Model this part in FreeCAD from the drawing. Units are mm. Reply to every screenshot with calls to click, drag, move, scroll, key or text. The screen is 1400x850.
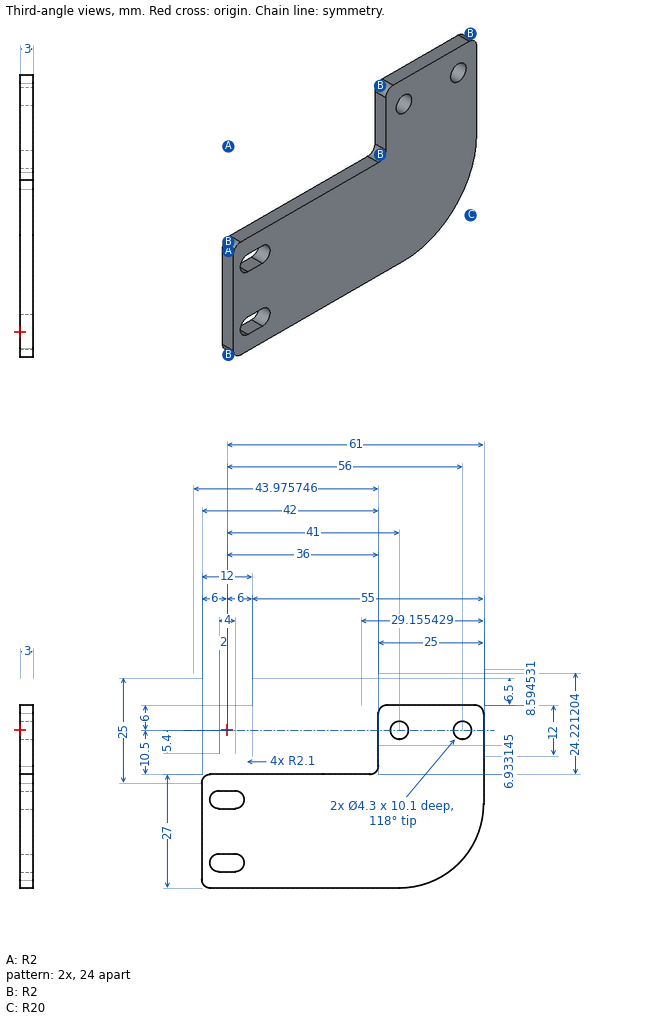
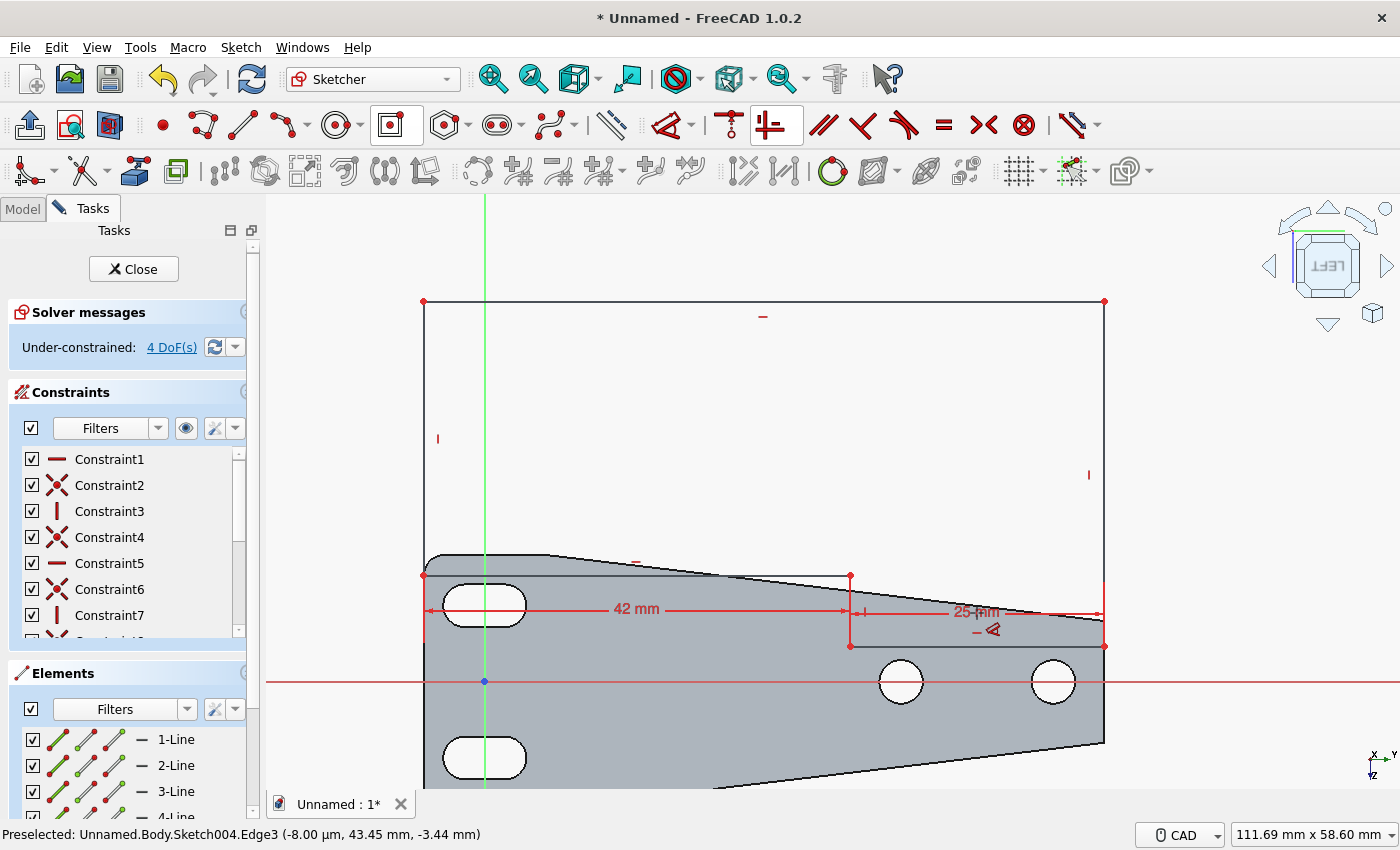
click(424, 384)
click(390, 439)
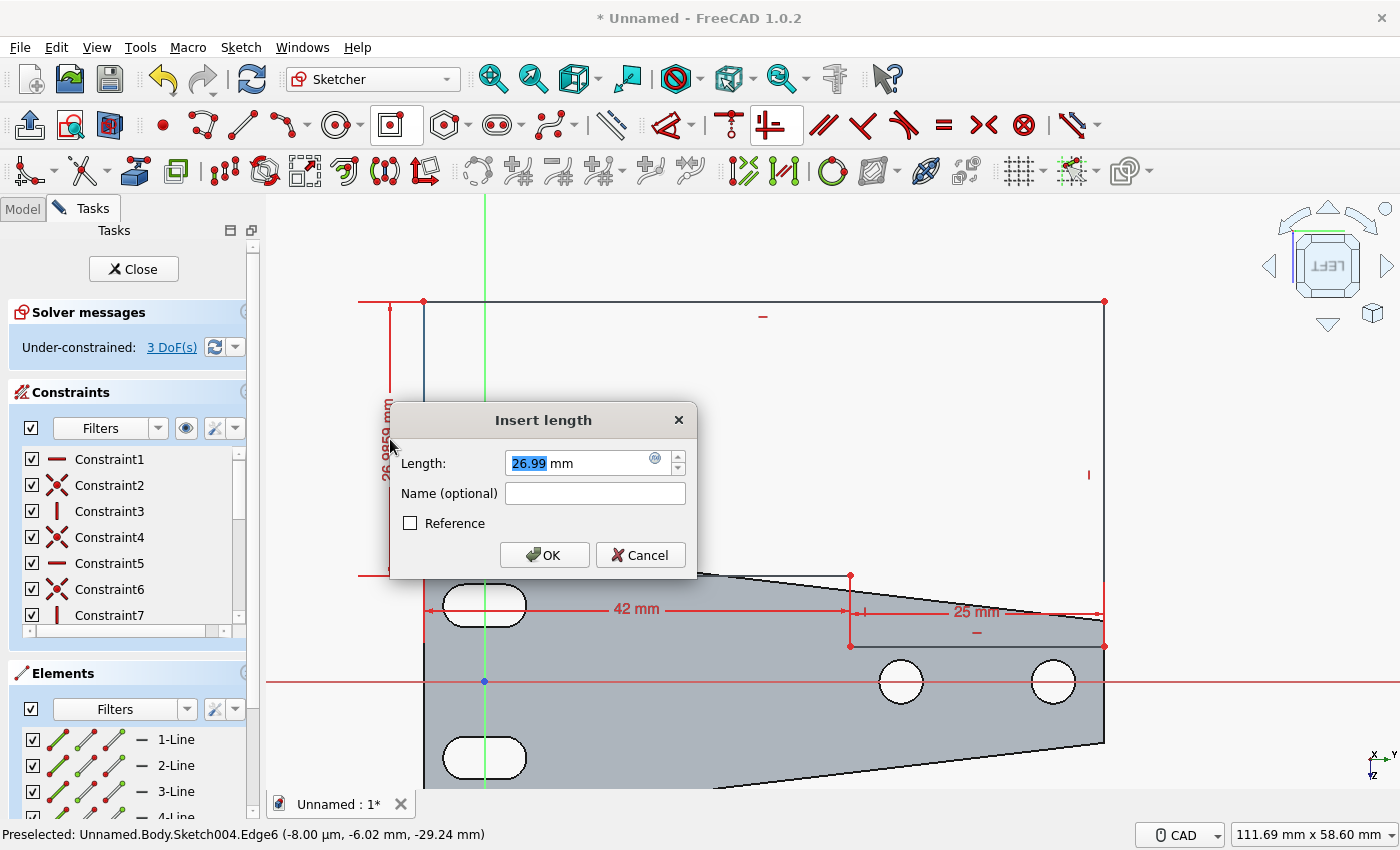
text(27)
key(Return)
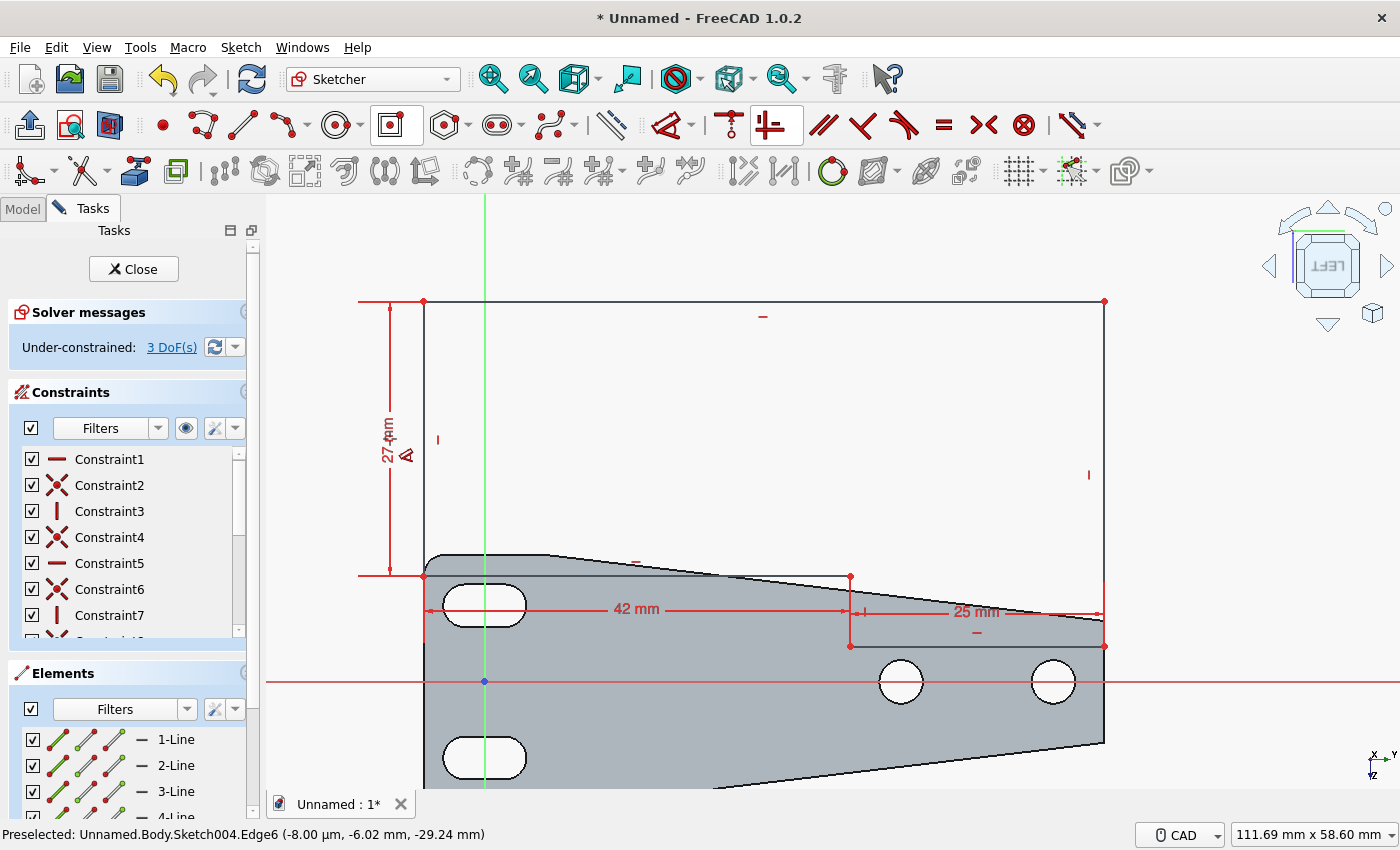
click(424, 576)
click(454, 716)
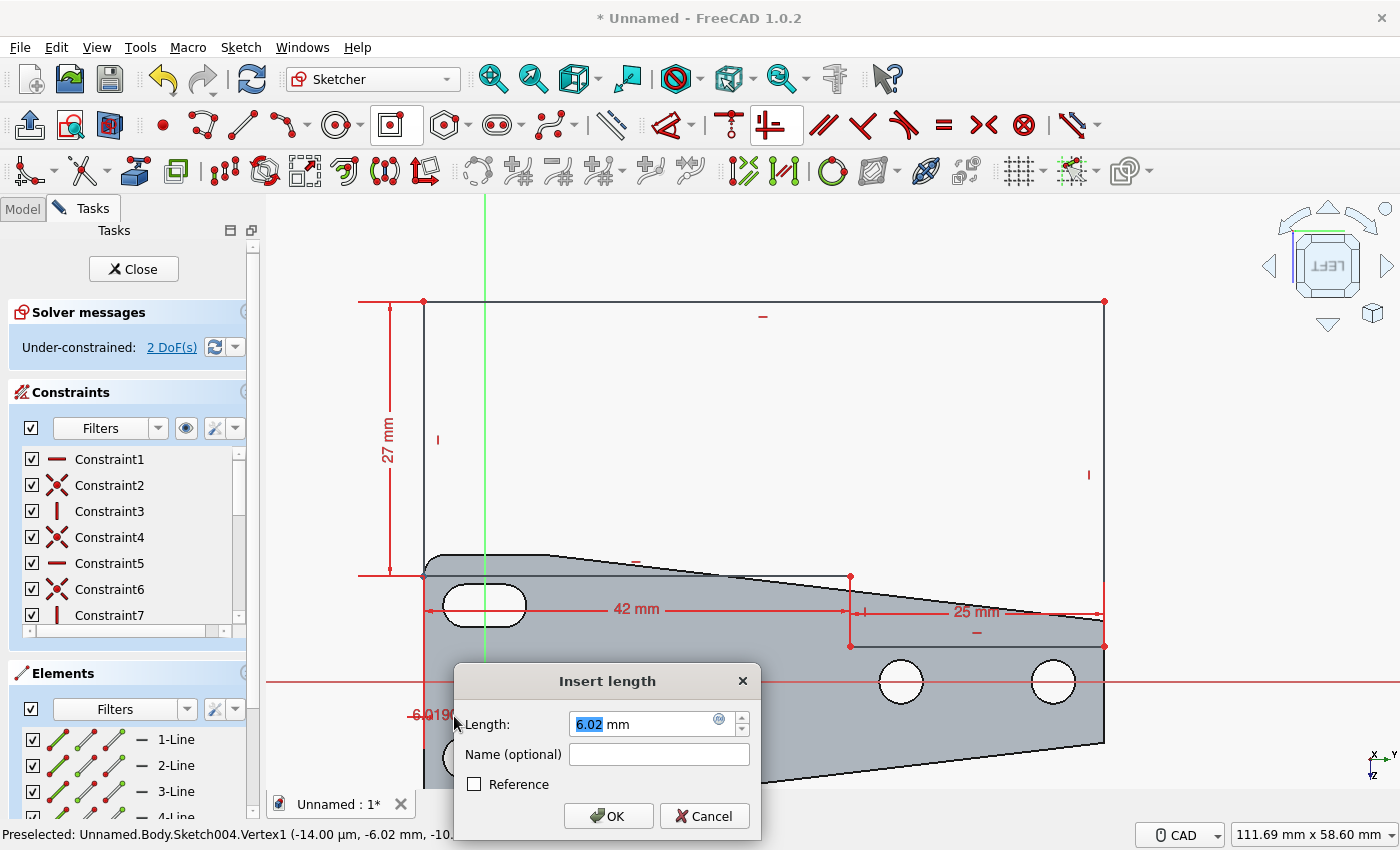
text(6)
key(Return)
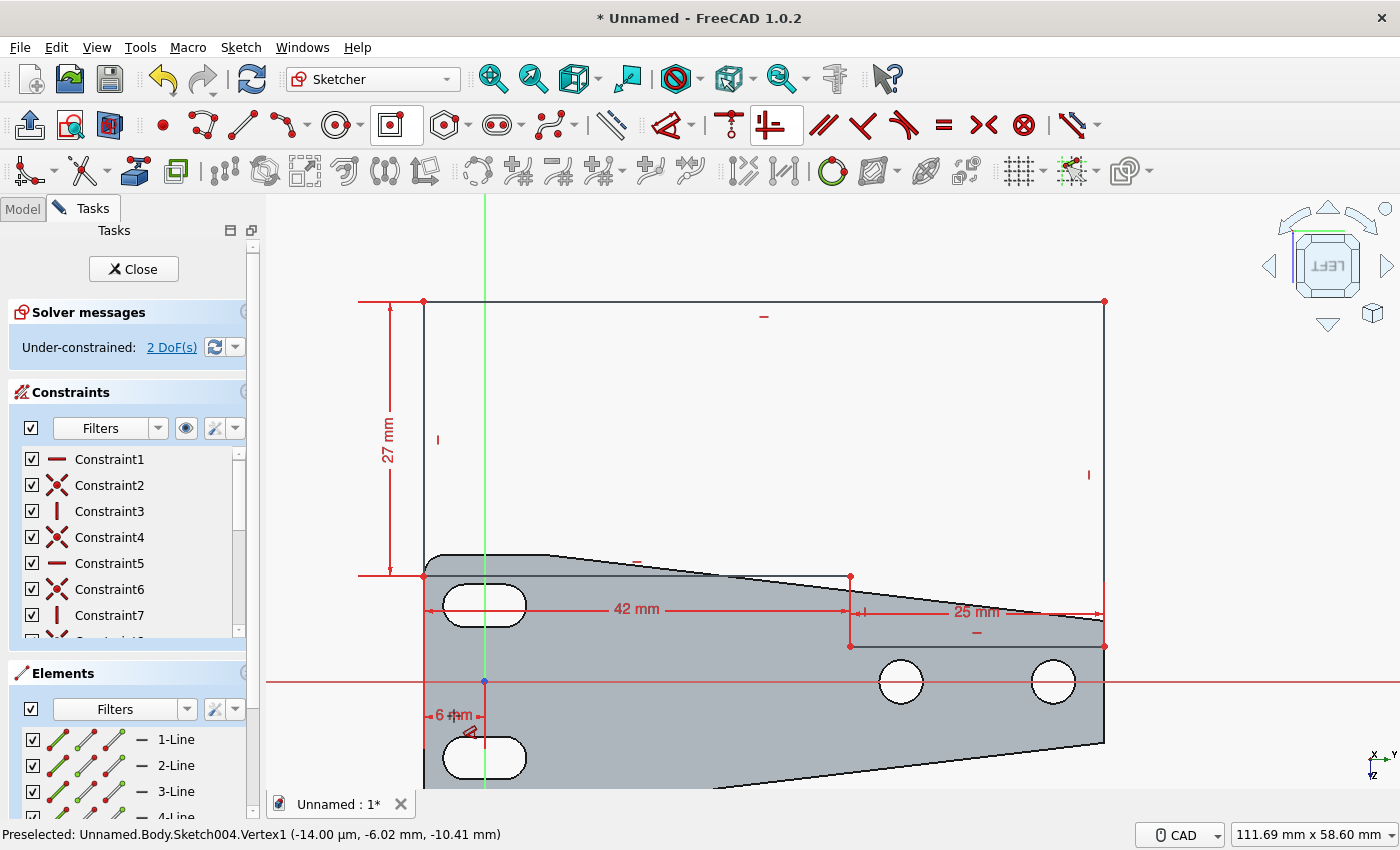
click(424, 576)
click(390, 629)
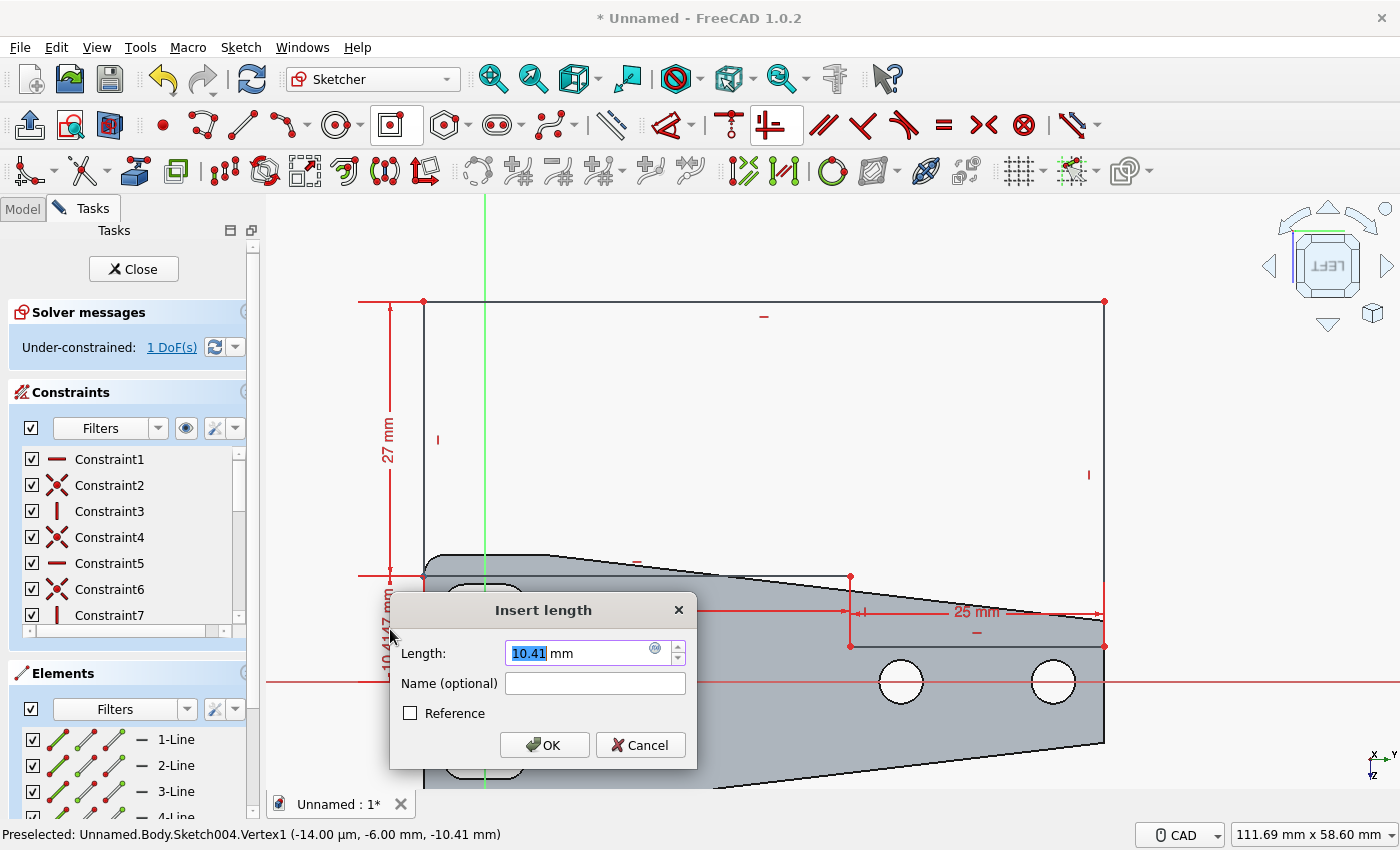
text(10.5)
key(Return)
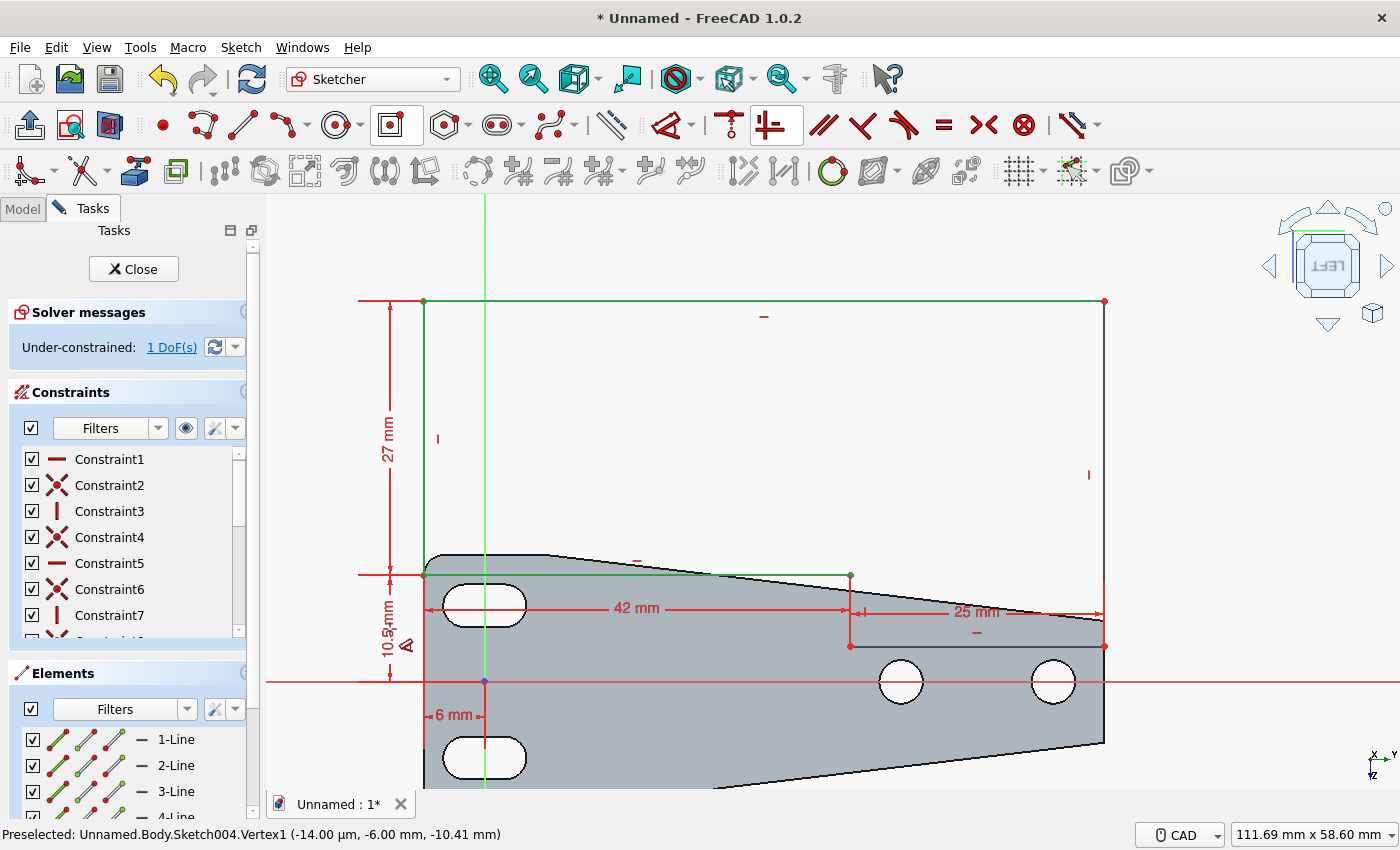
click(850, 597)
click(884, 611)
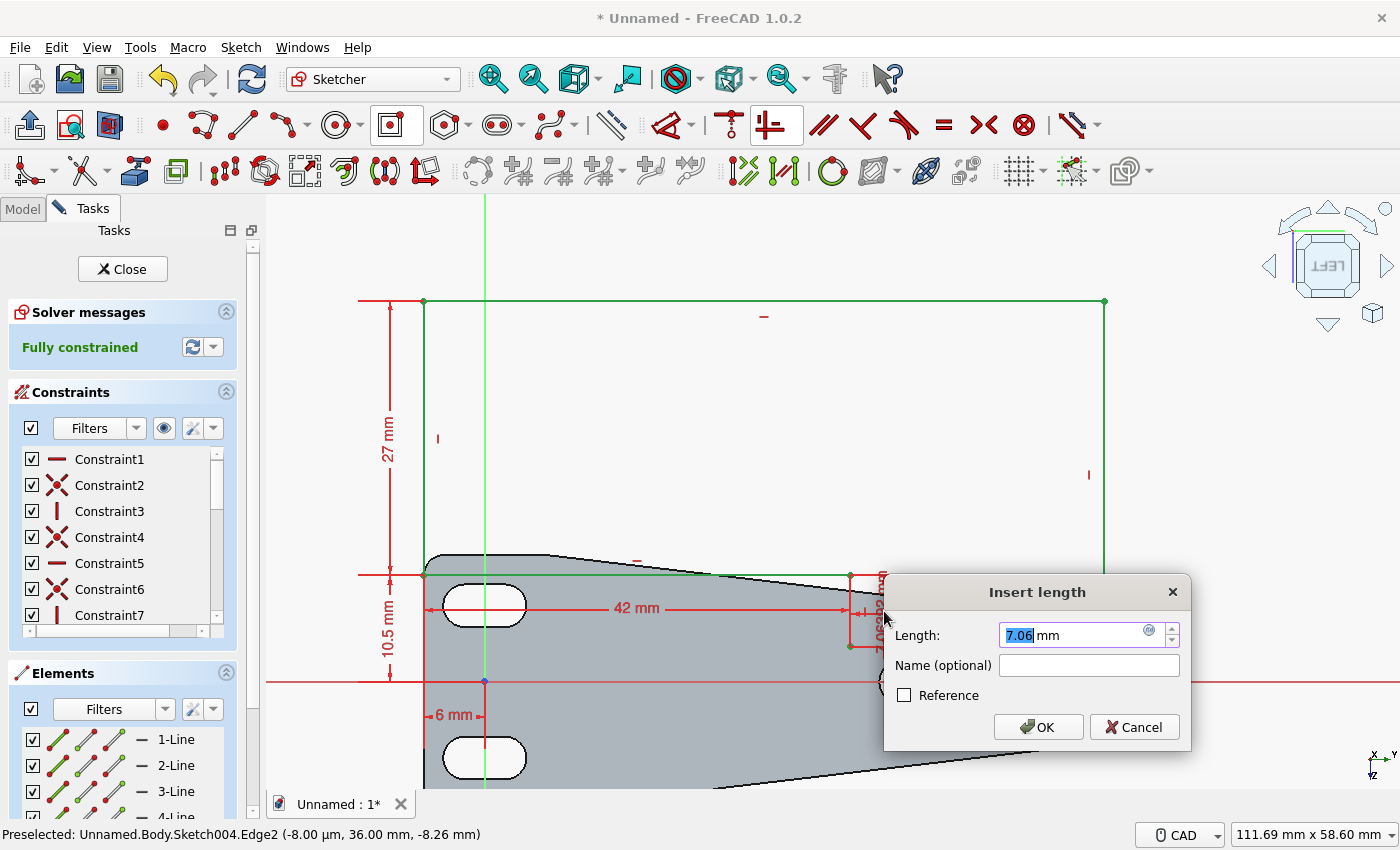
text(6.933145)
key(Return)
key(Escape)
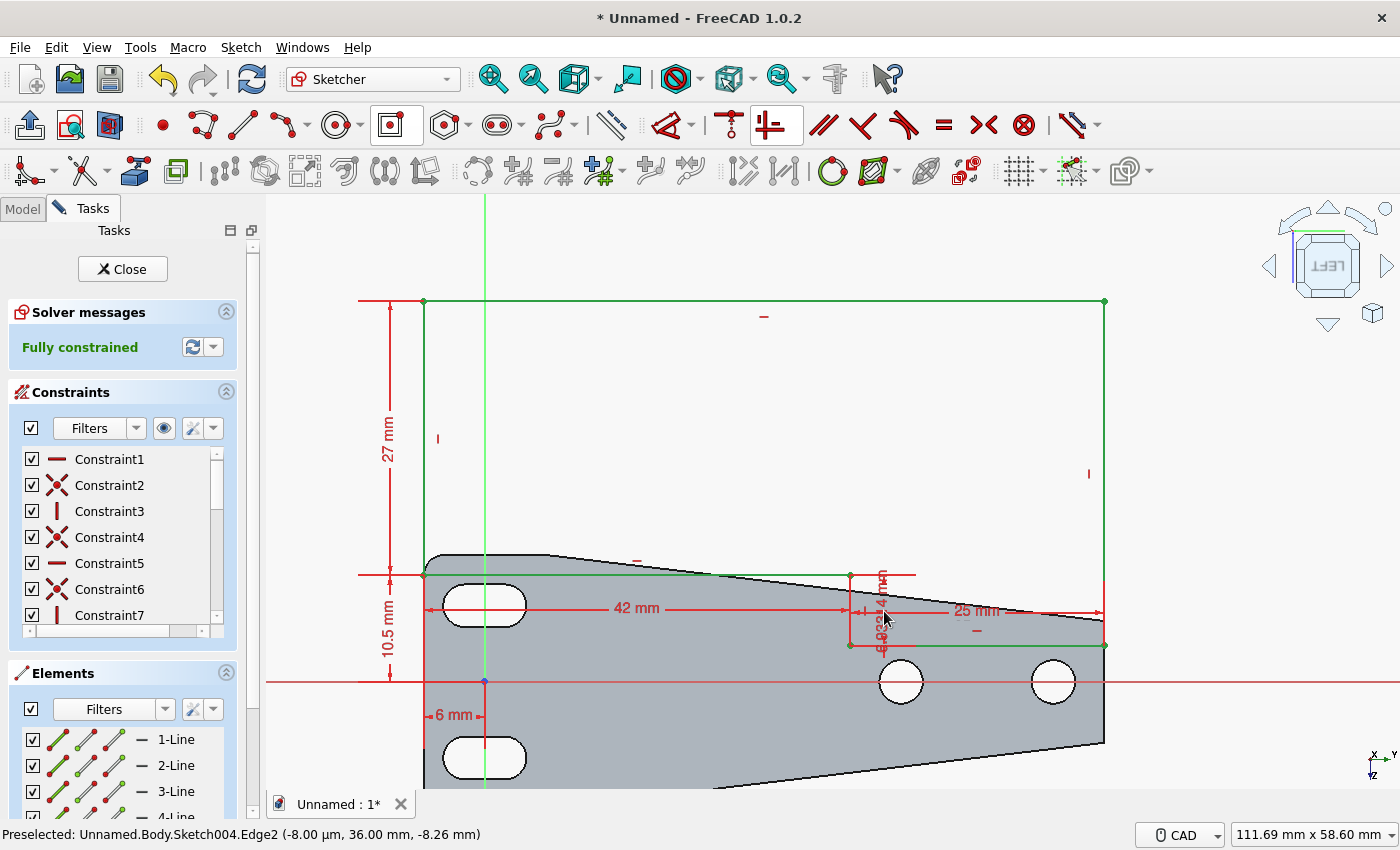
click(123, 269)